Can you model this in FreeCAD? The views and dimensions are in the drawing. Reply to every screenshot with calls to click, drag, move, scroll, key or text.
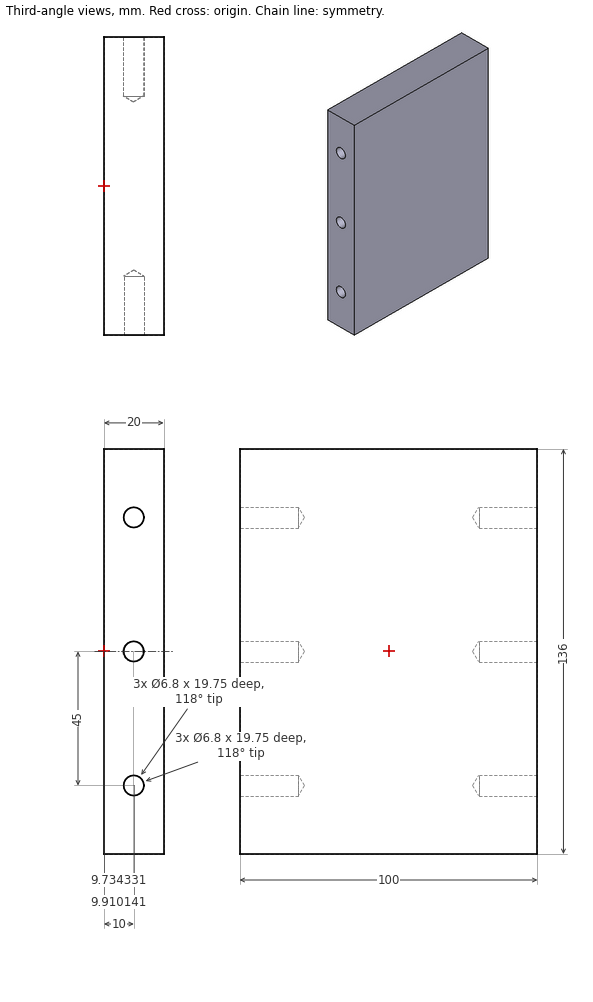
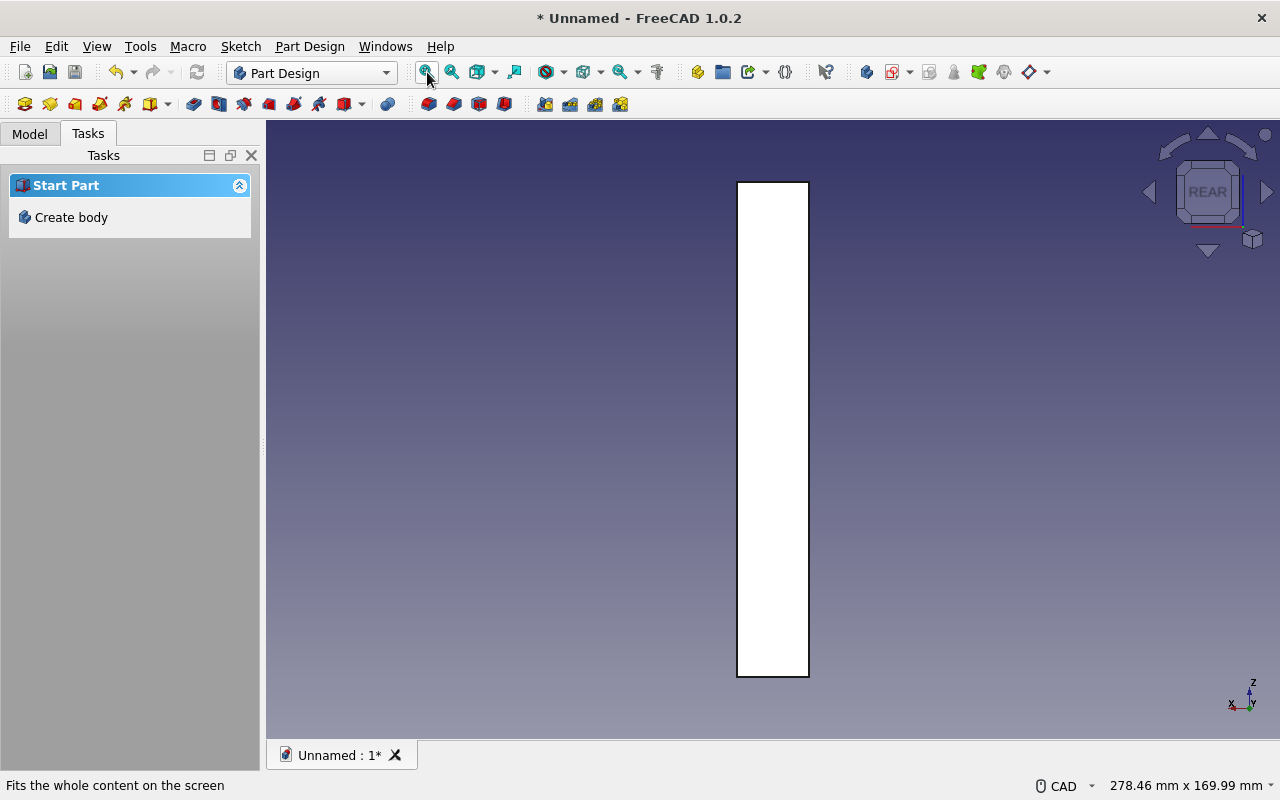
click(773, 429)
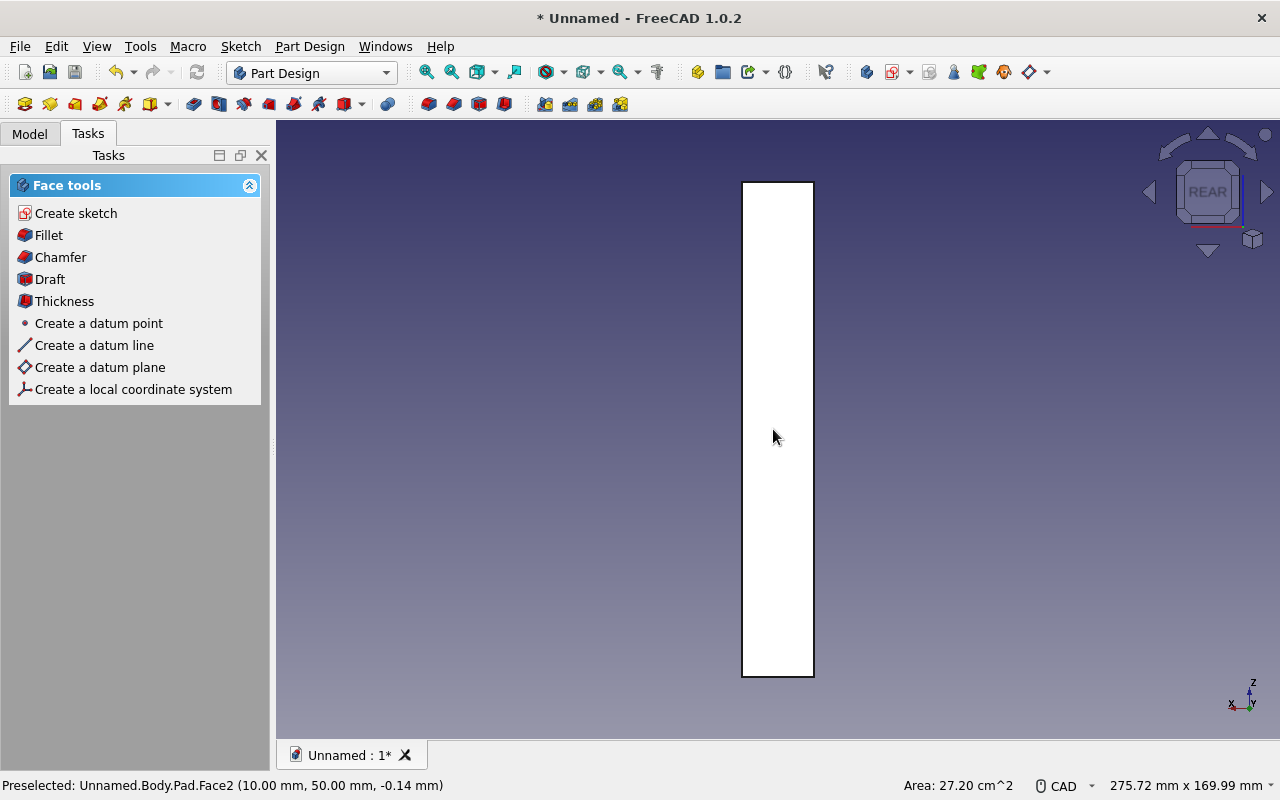
click(892, 72)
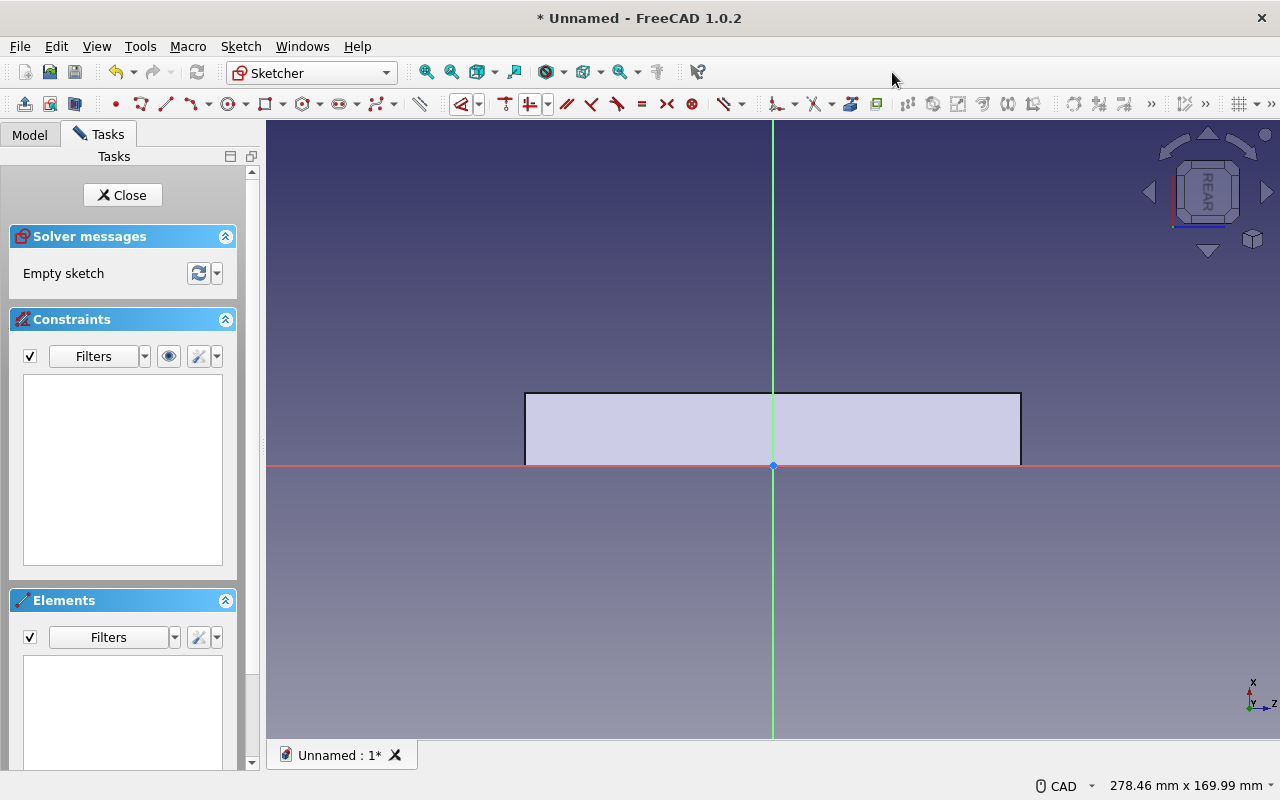
scroll(912, 466, up, 2)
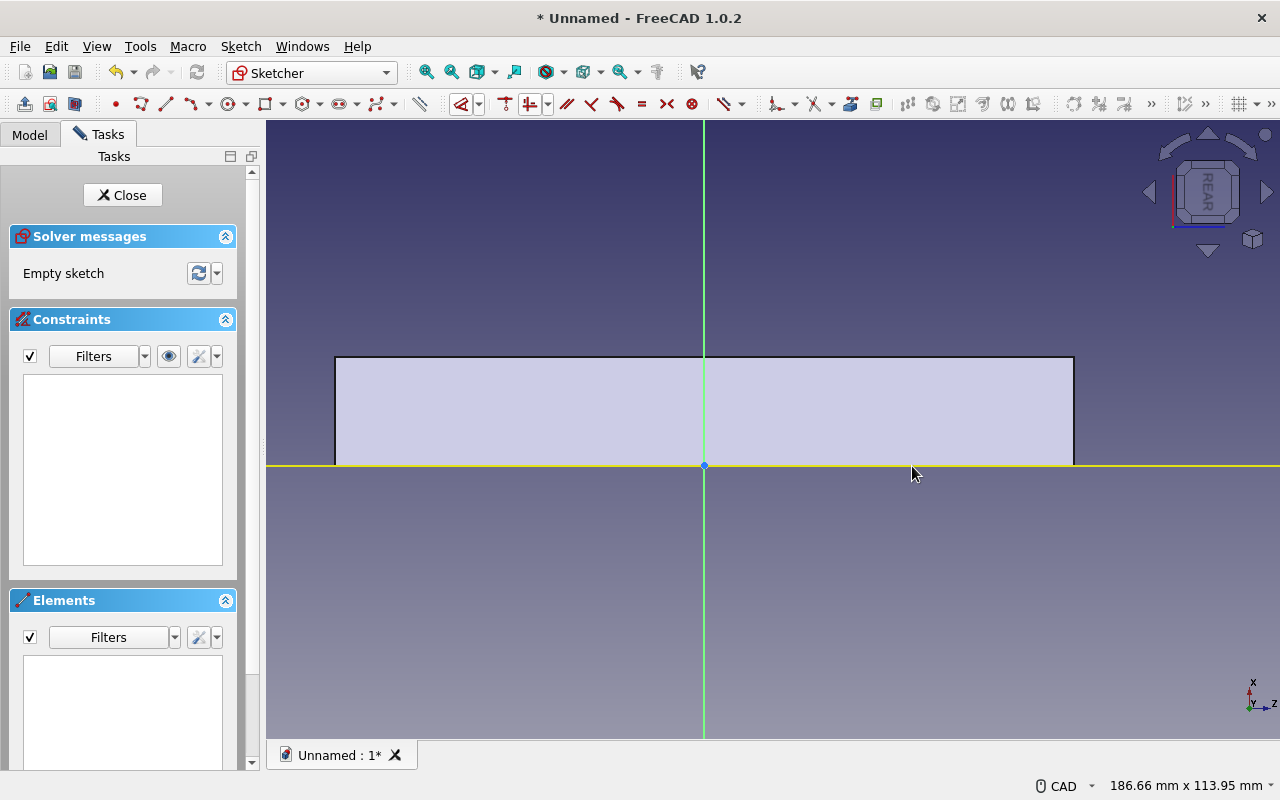
click(228, 104)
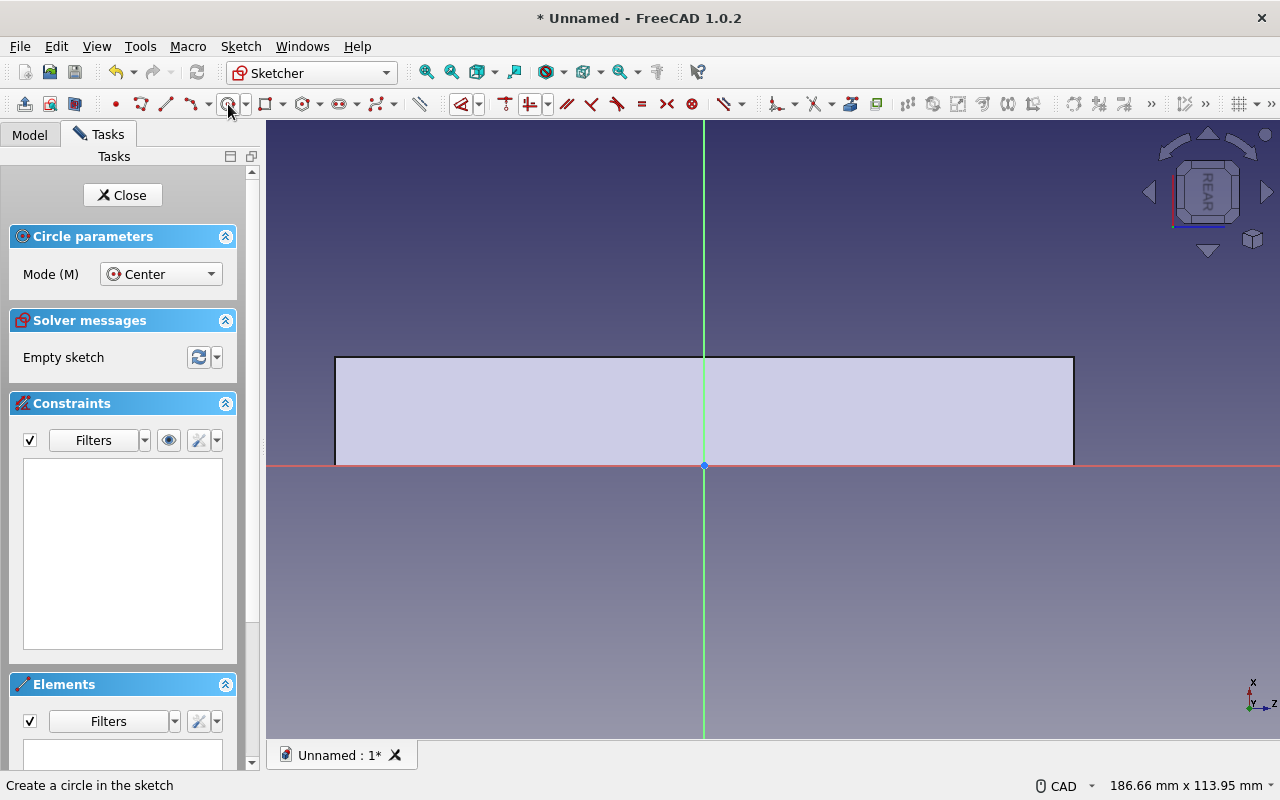
scroll(460, 412, up, 2)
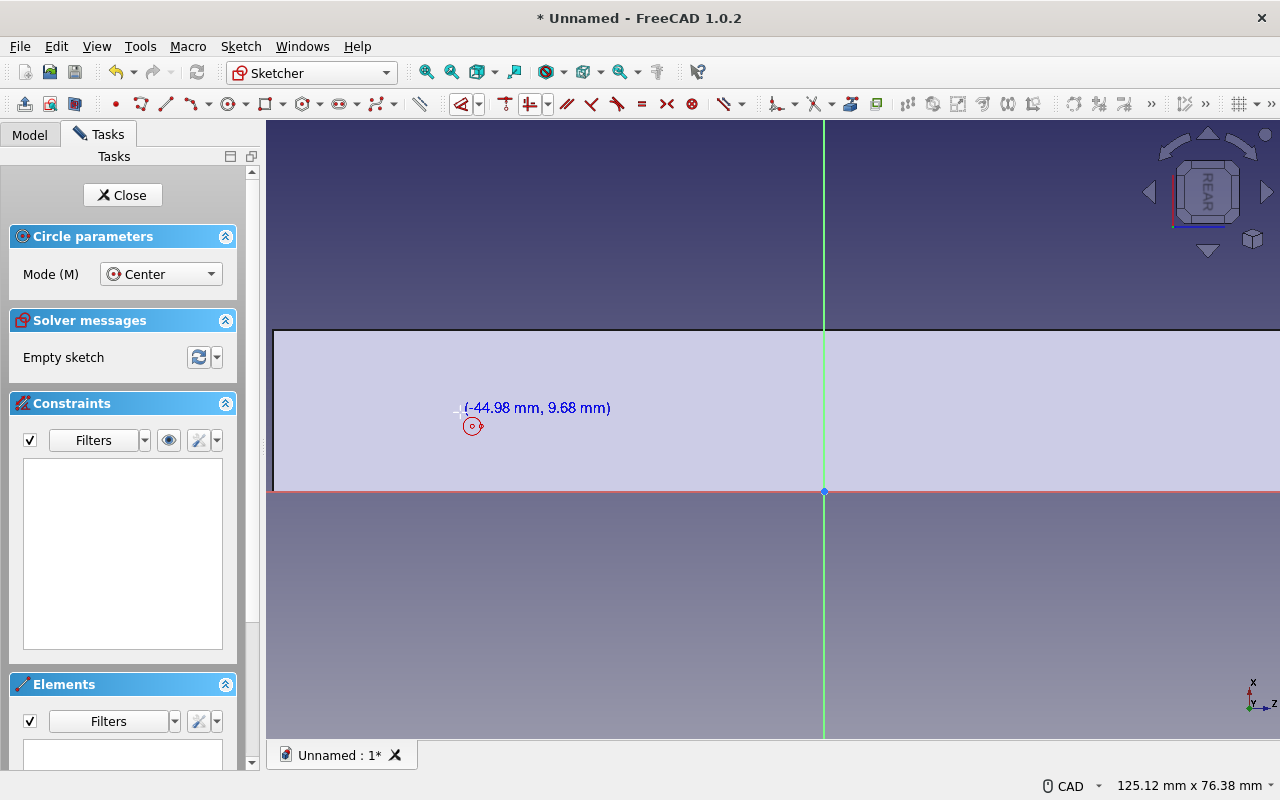
click(460, 411)
click(479, 392)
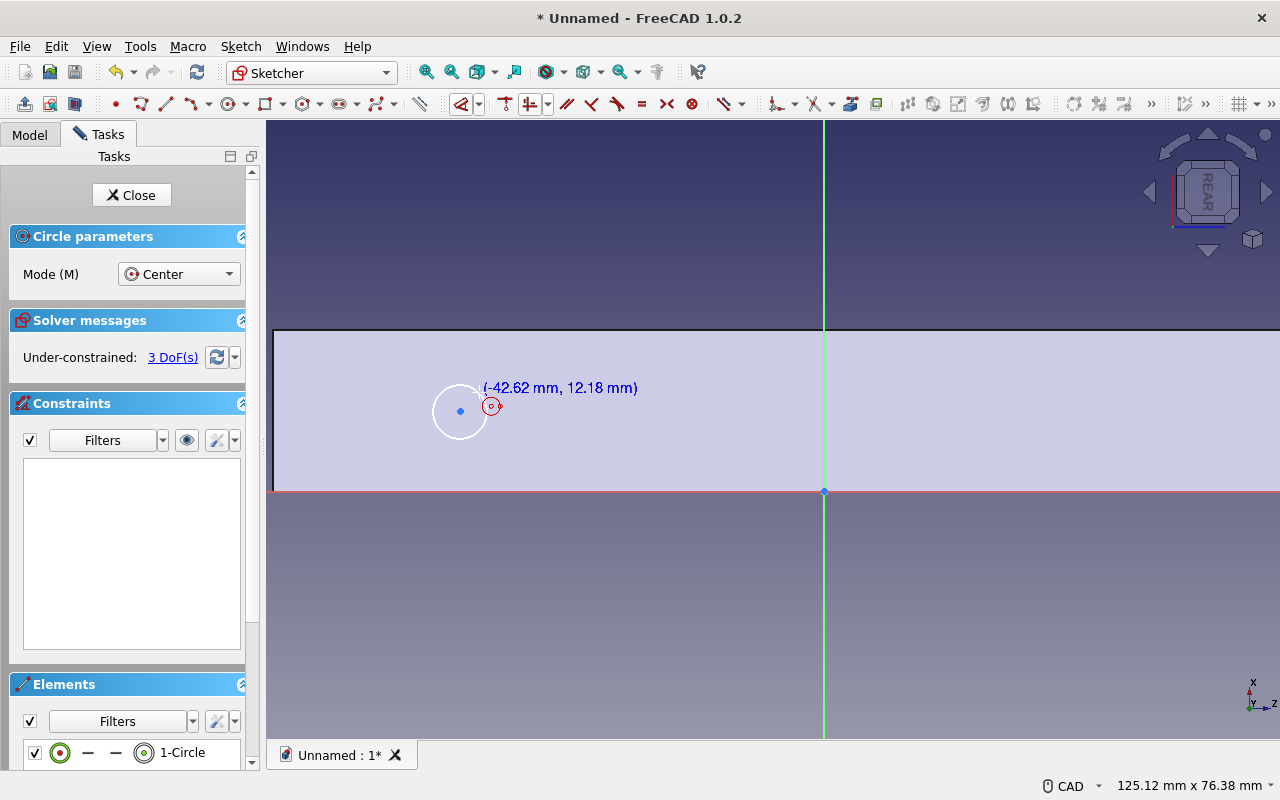
scroll(461, 413, down, 2)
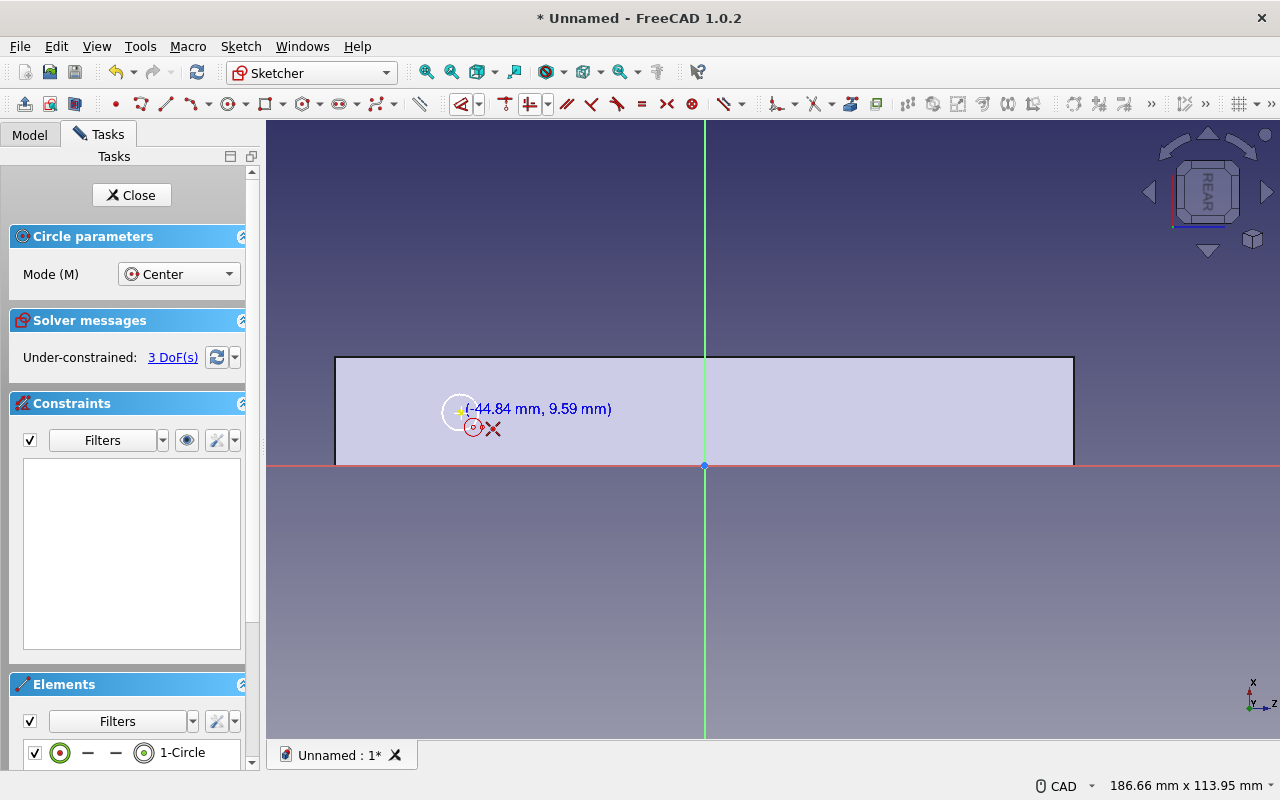
scroll(949, 412, up, 2)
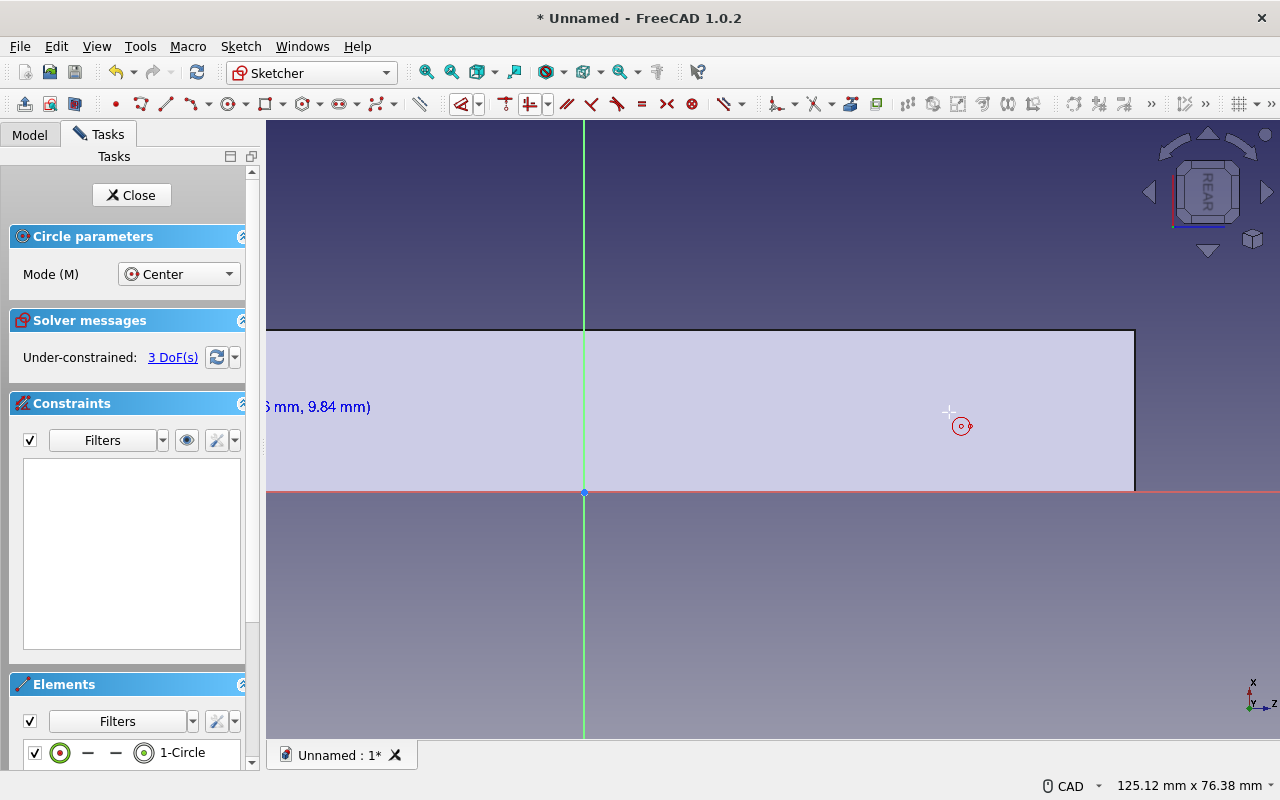
click(949, 412)
click(968, 392)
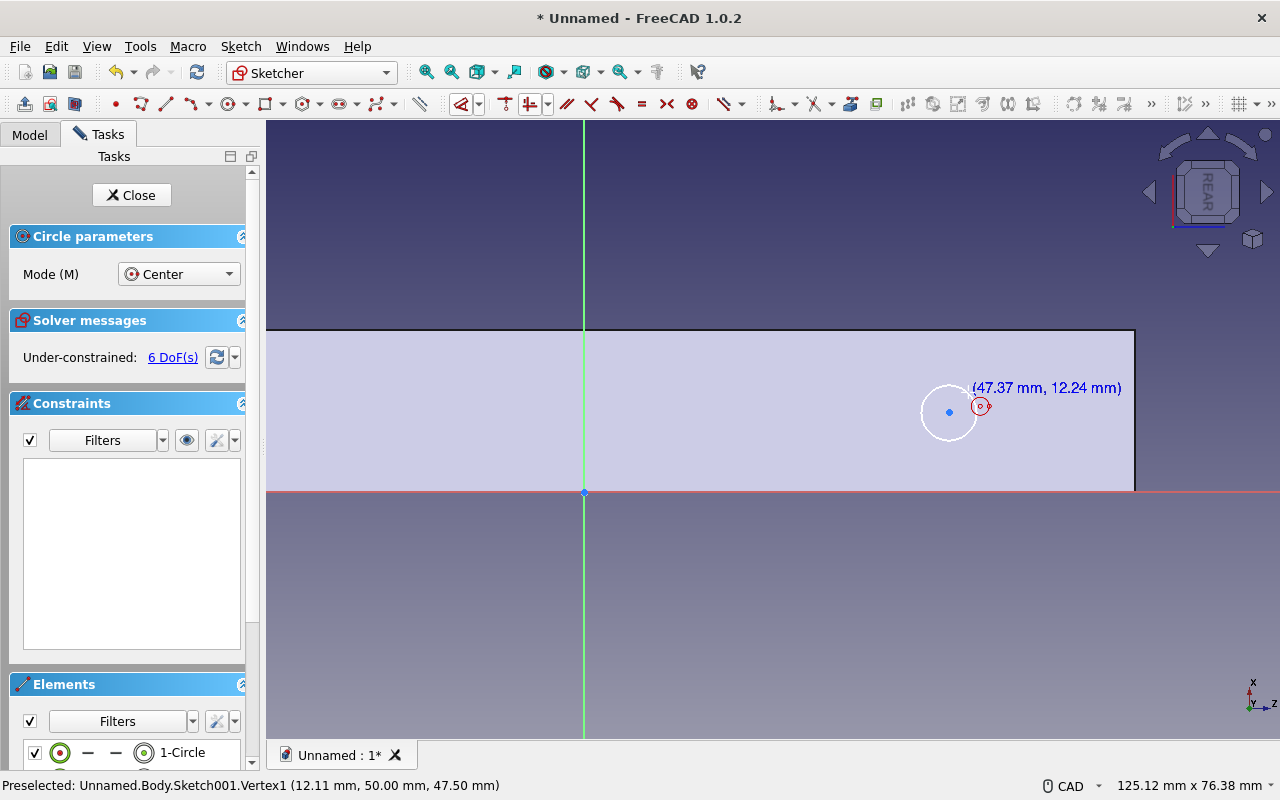
click(584, 413)
click(604, 394)
key(Escape)